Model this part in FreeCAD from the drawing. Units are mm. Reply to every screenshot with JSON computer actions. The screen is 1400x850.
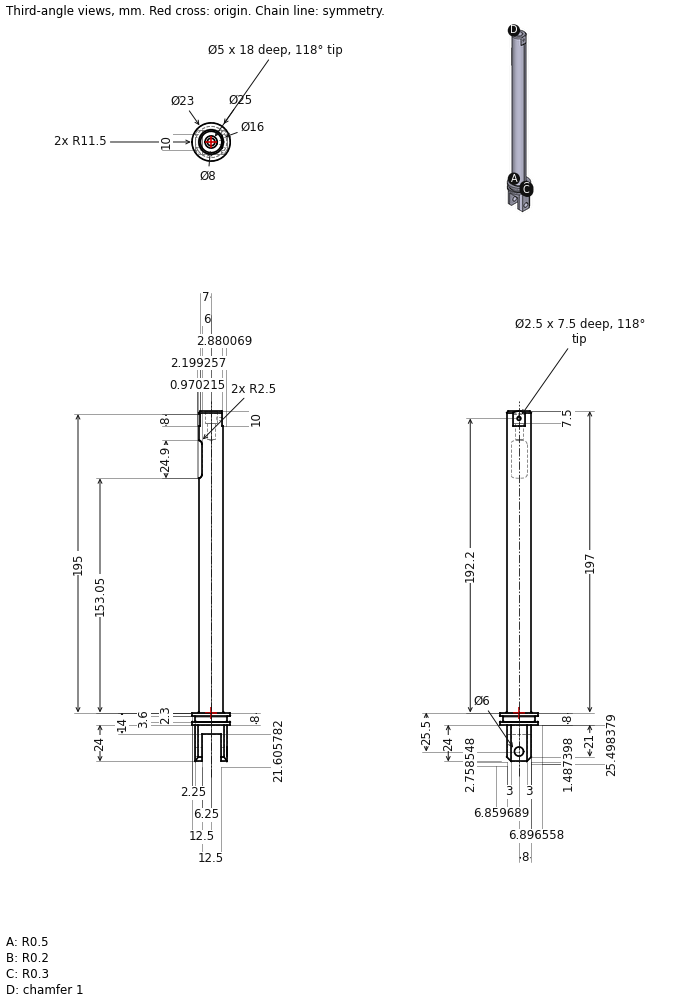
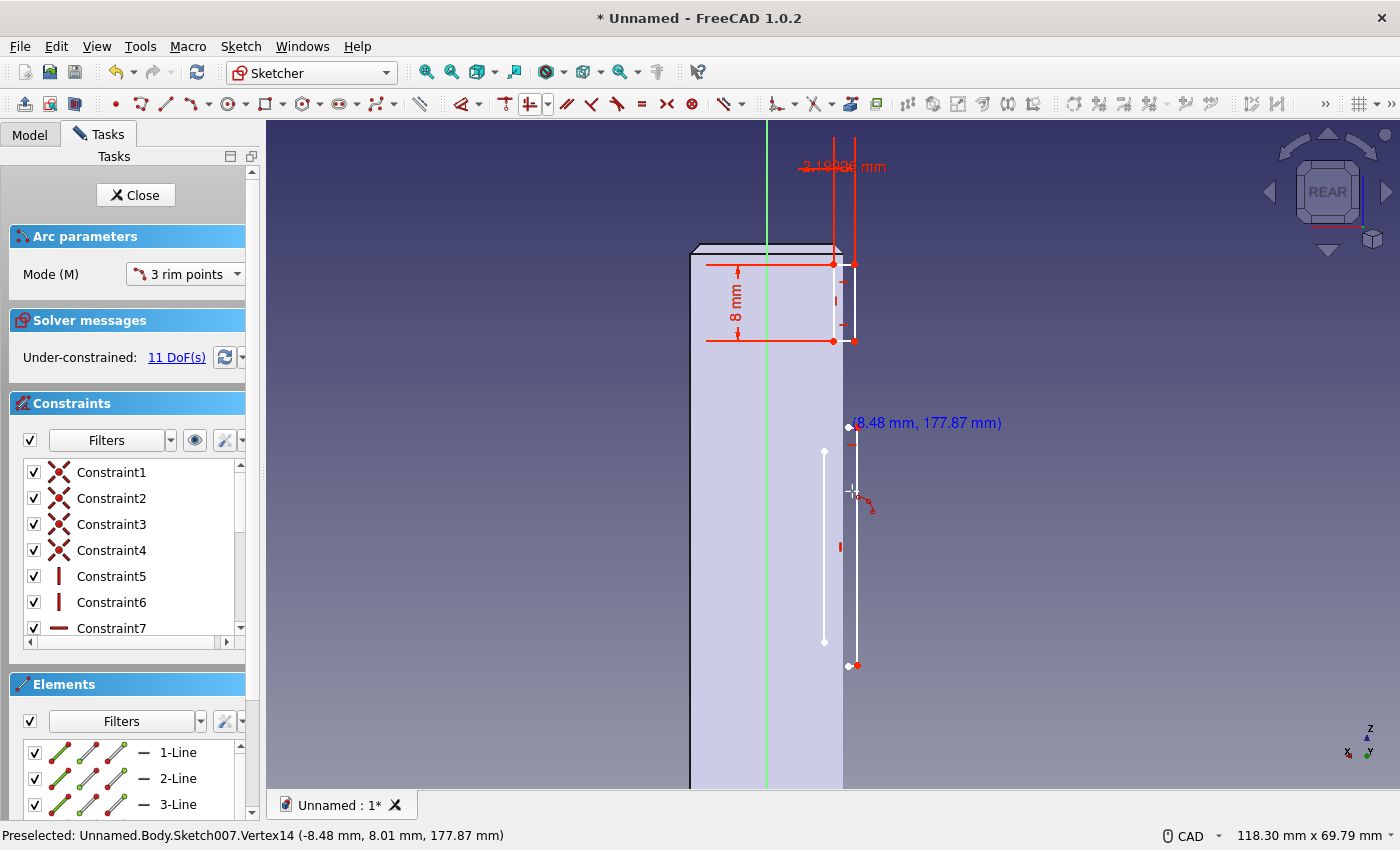
{"action": "left_click", "coordinate": [824, 451]}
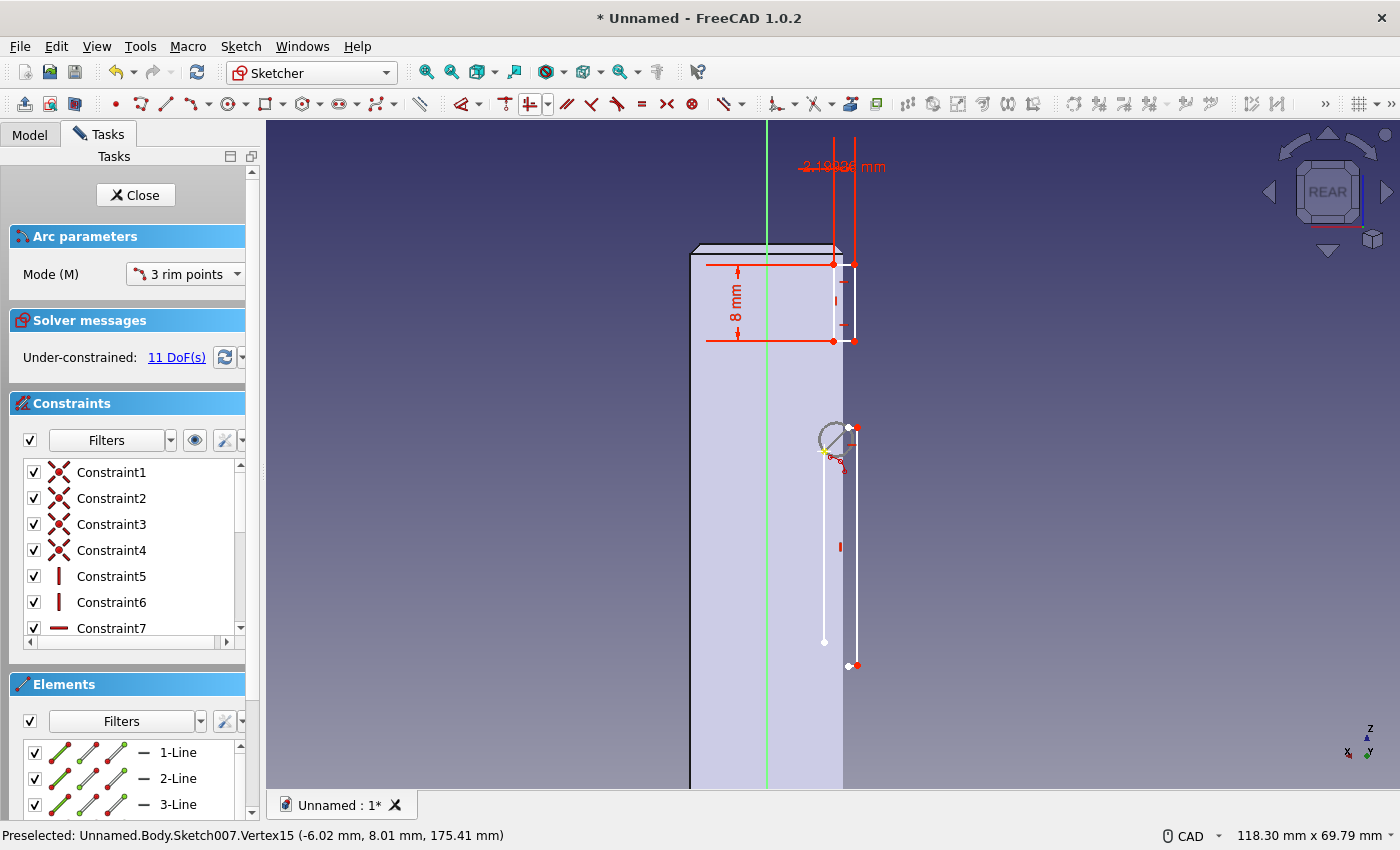
{"action": "scroll", "coordinate": [831, 434], "scroll_direction": "up", "scroll_amount": 5}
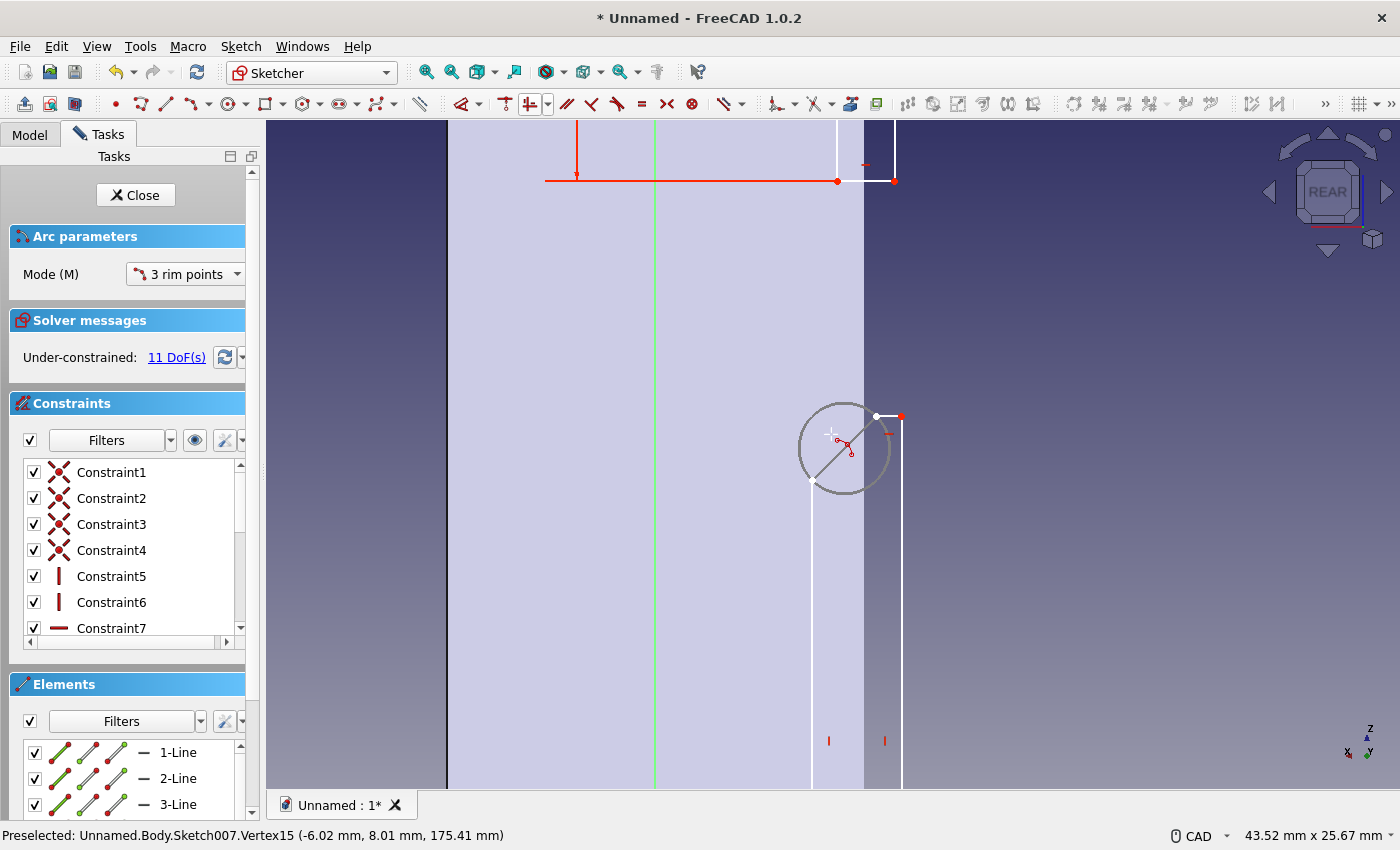
{"action": "left_click", "coordinate": [831, 433]}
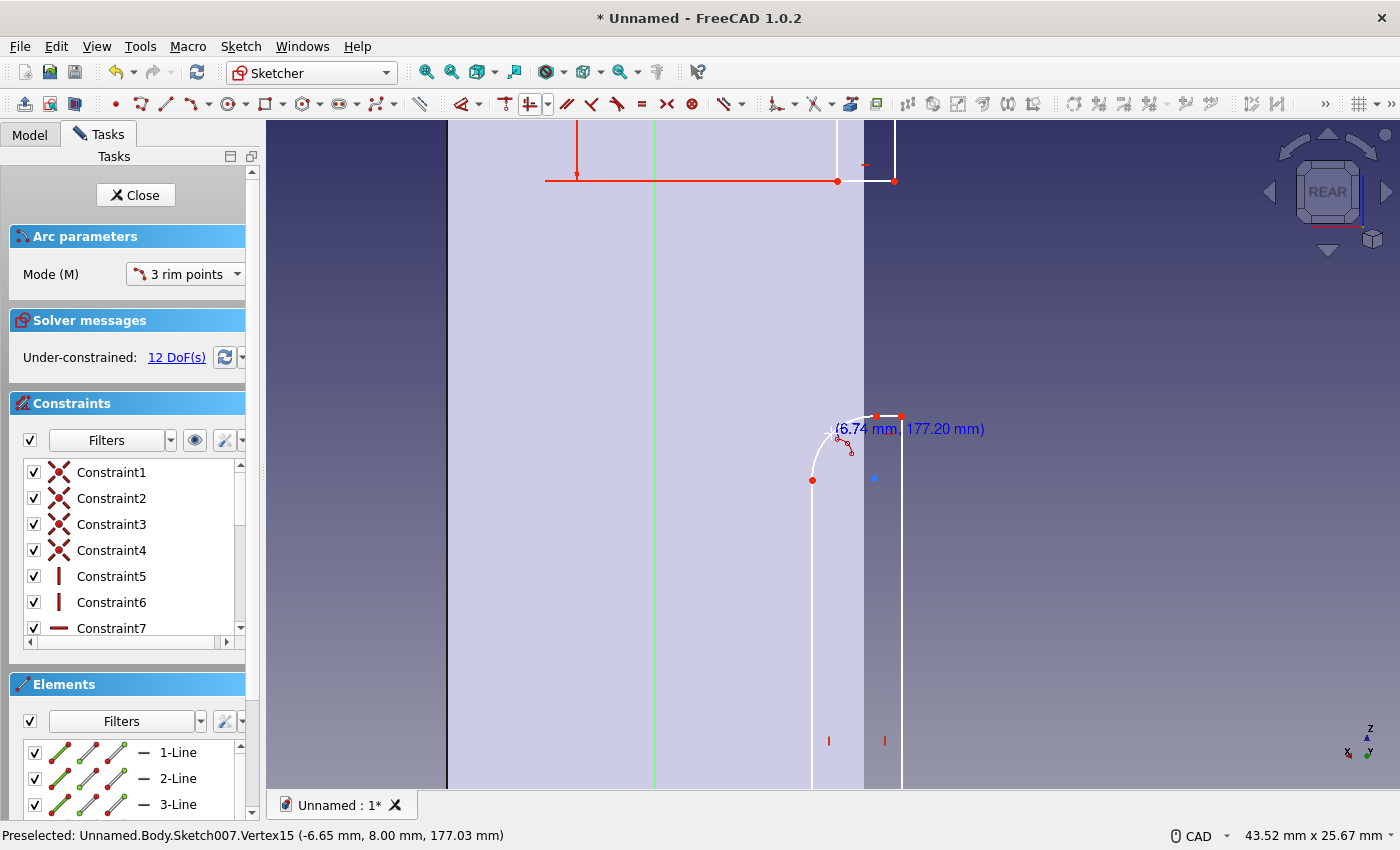
{"action": "scroll", "coordinate": [831, 433], "scroll_direction": "down", "scroll_amount": 5}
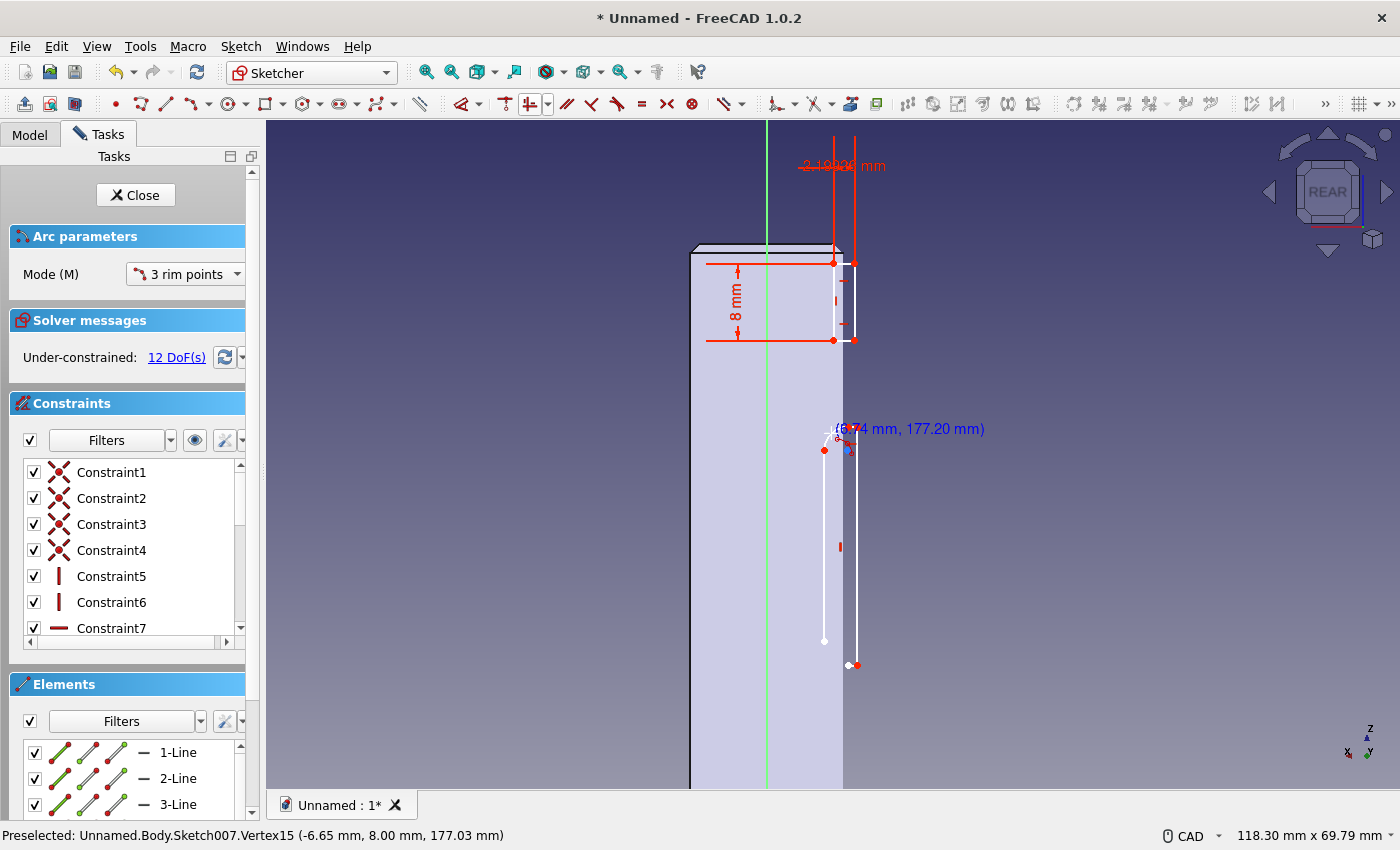
{"action": "left_click", "coordinate": [824, 642]}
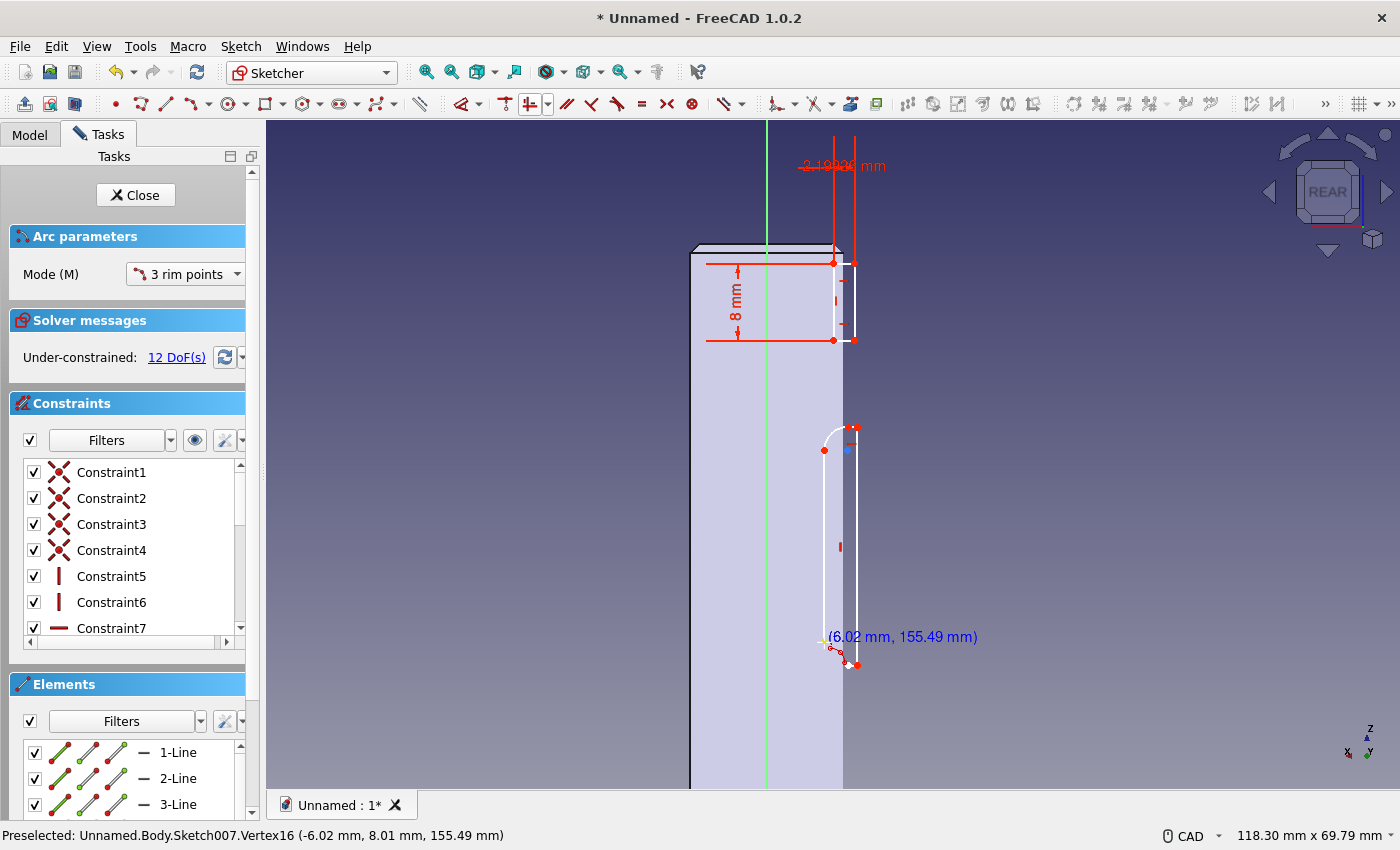
{"action": "scroll", "coordinate": [848, 665], "scroll_direction": "up", "scroll_amount": 7}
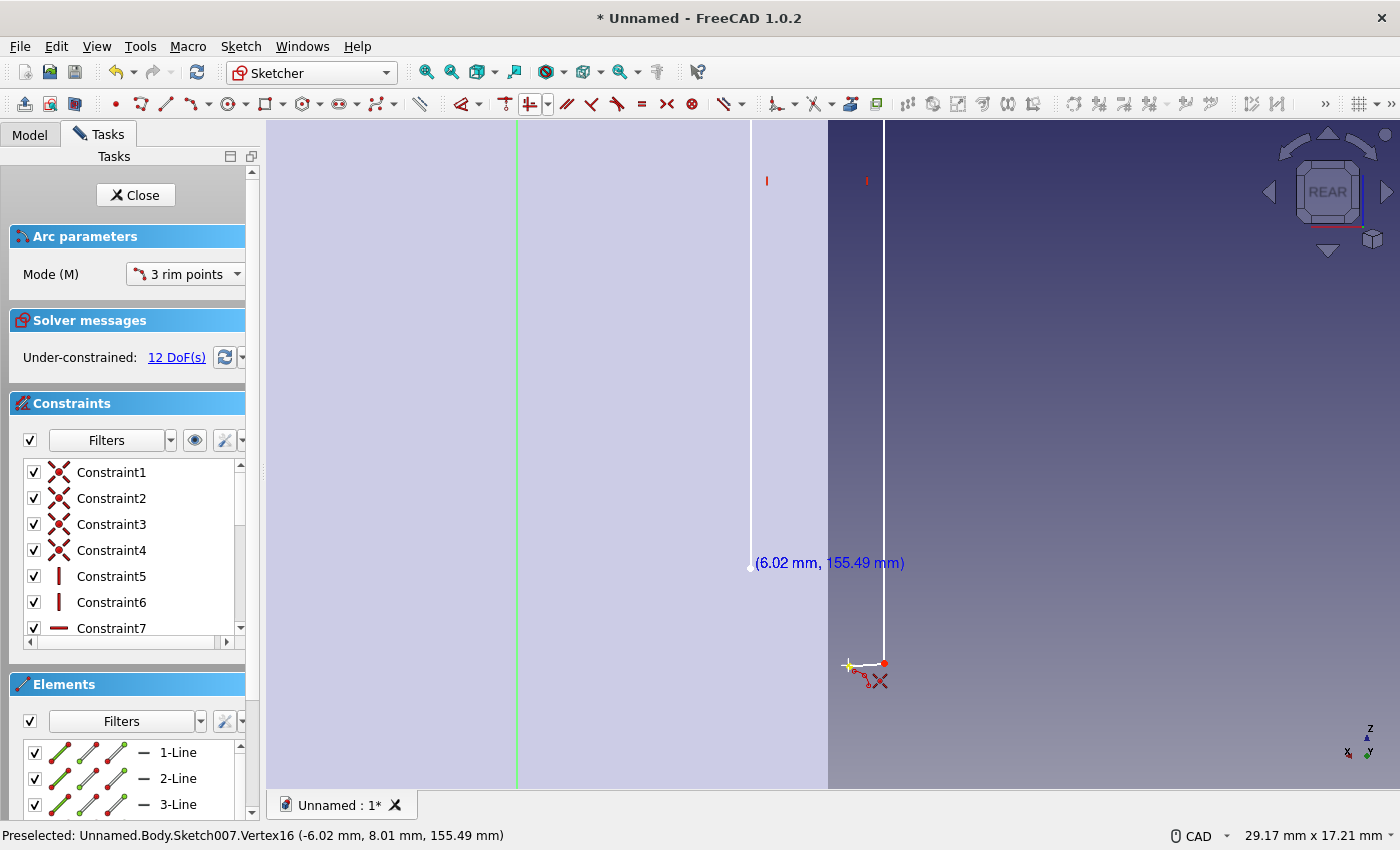
{"action": "left_click", "coordinate": [849, 666]}
{"action": "left_click", "coordinate": [779, 635]}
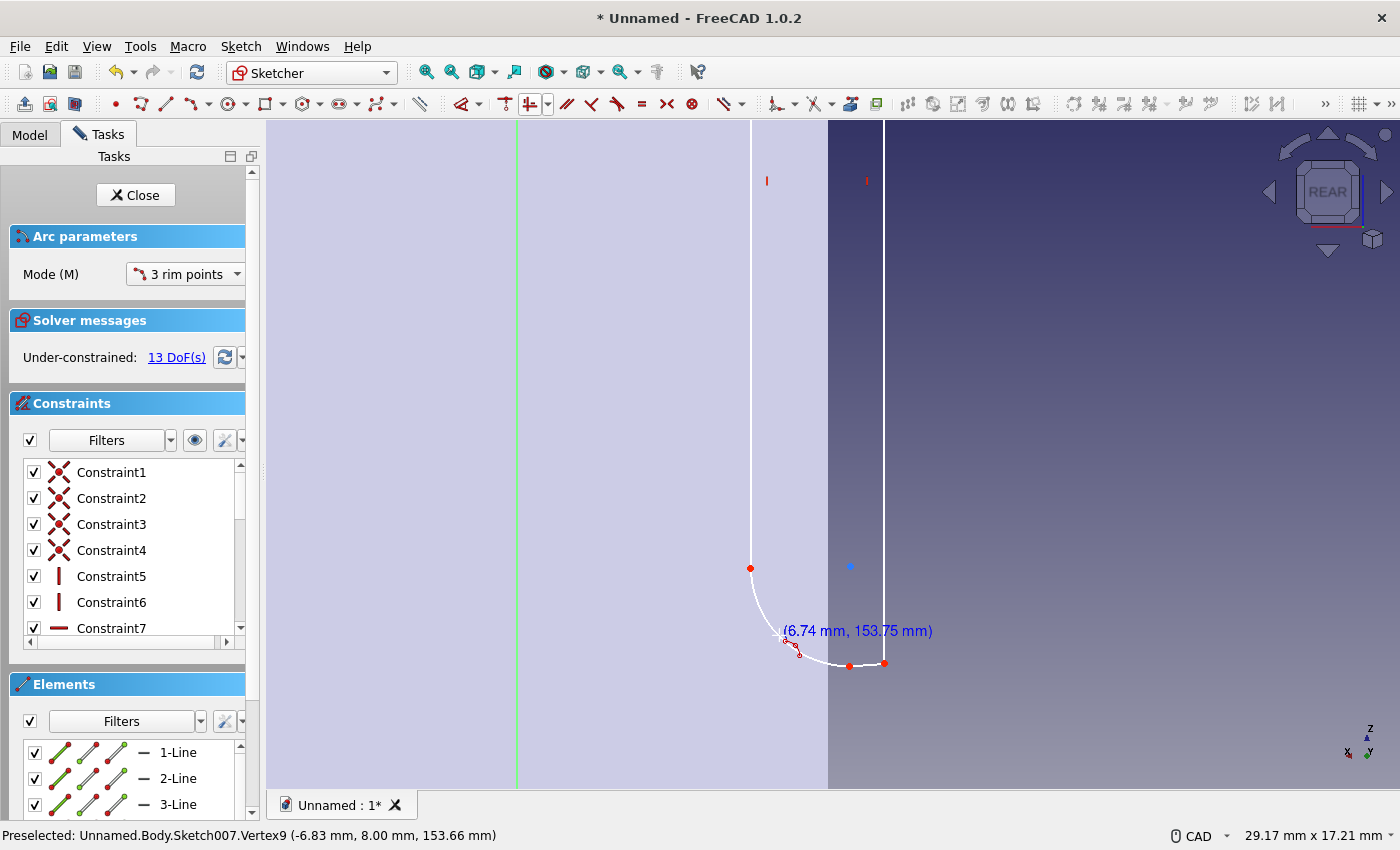
{"action": "left_click", "coordinate": [264, 104]}